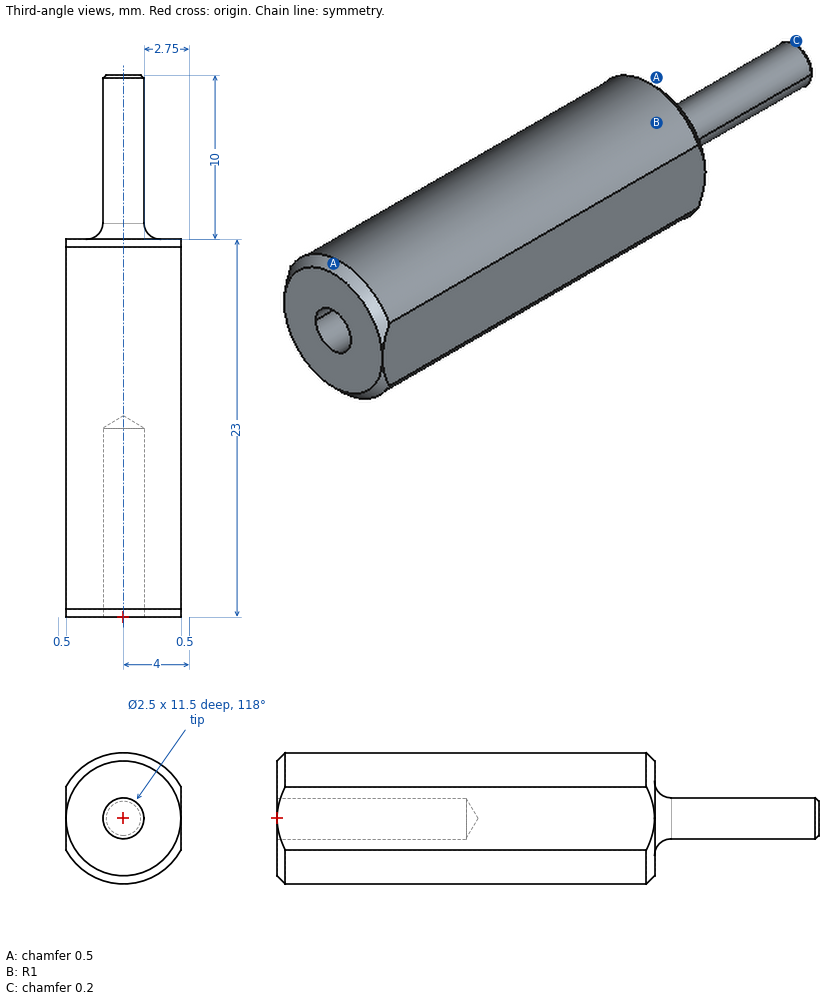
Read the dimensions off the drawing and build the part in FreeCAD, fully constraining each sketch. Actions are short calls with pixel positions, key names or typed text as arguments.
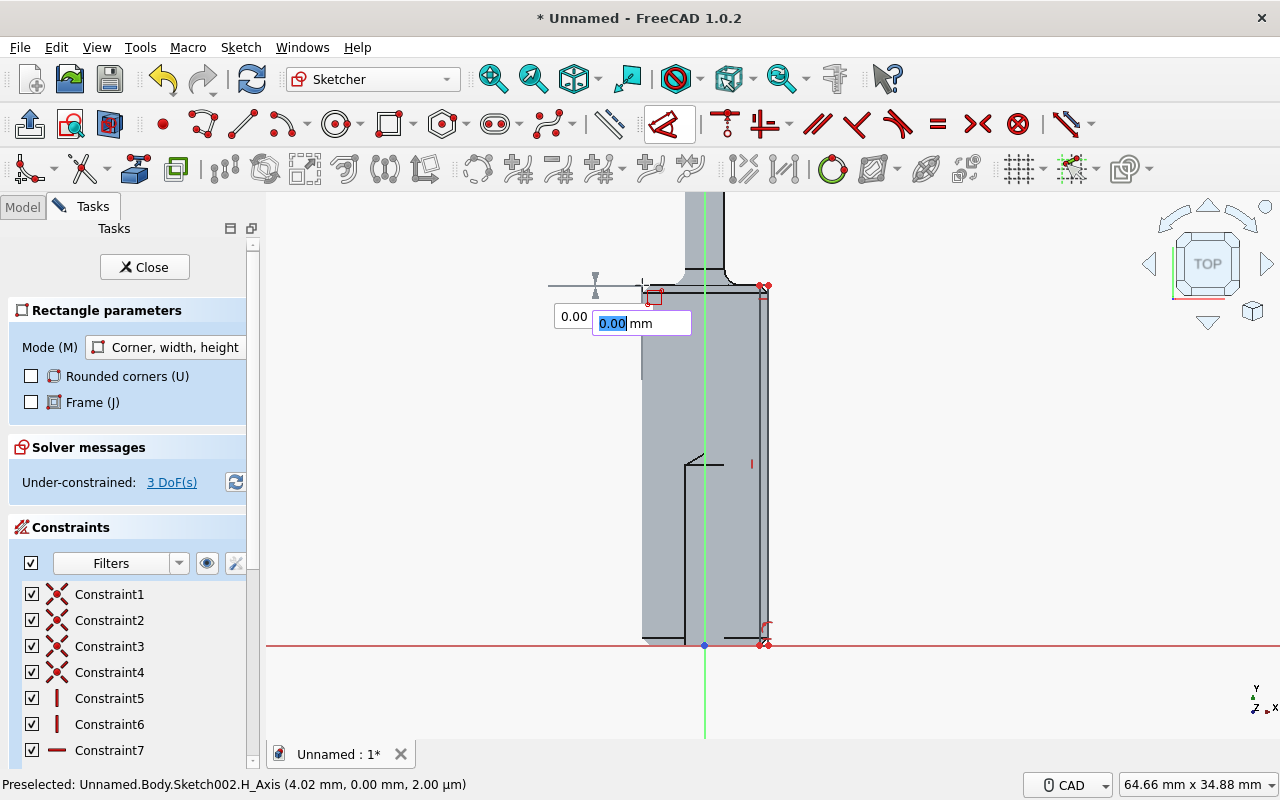
click(650, 646)
key(Escape)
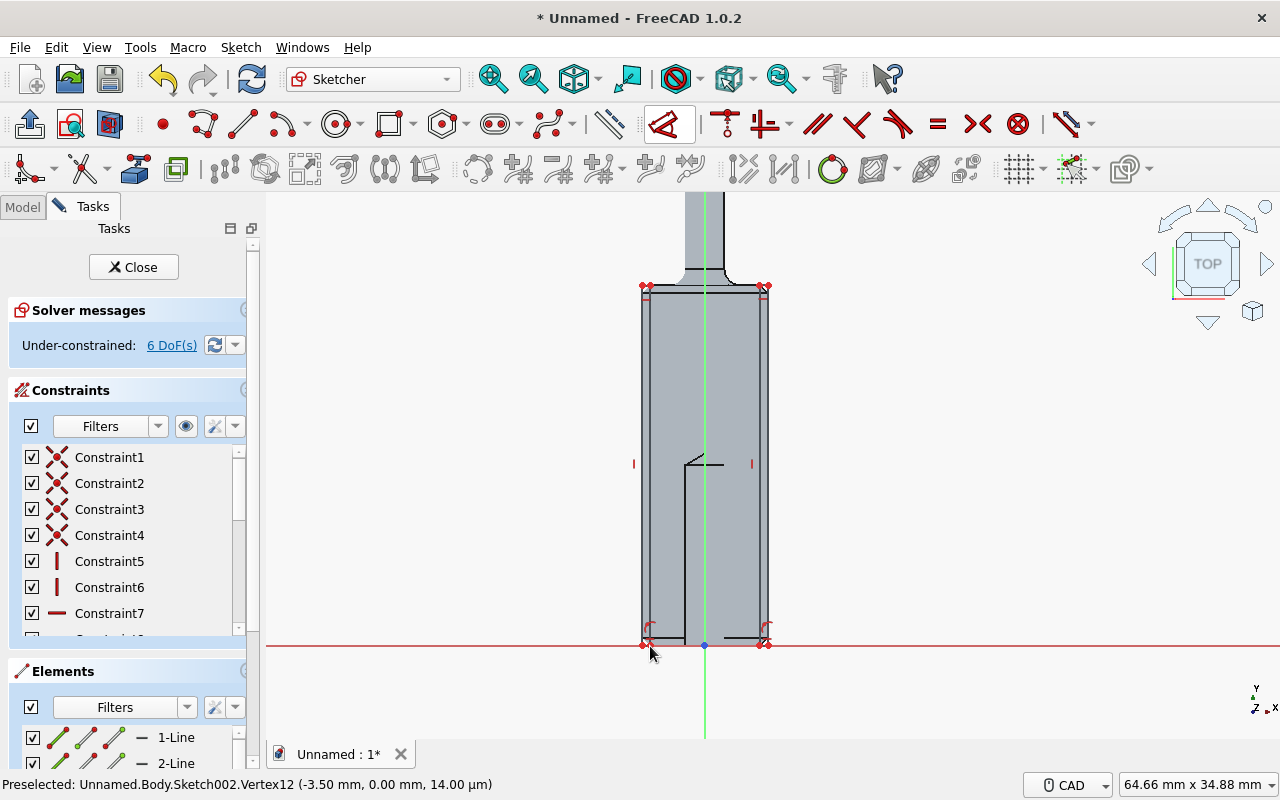
scroll(768, 285, up, 3)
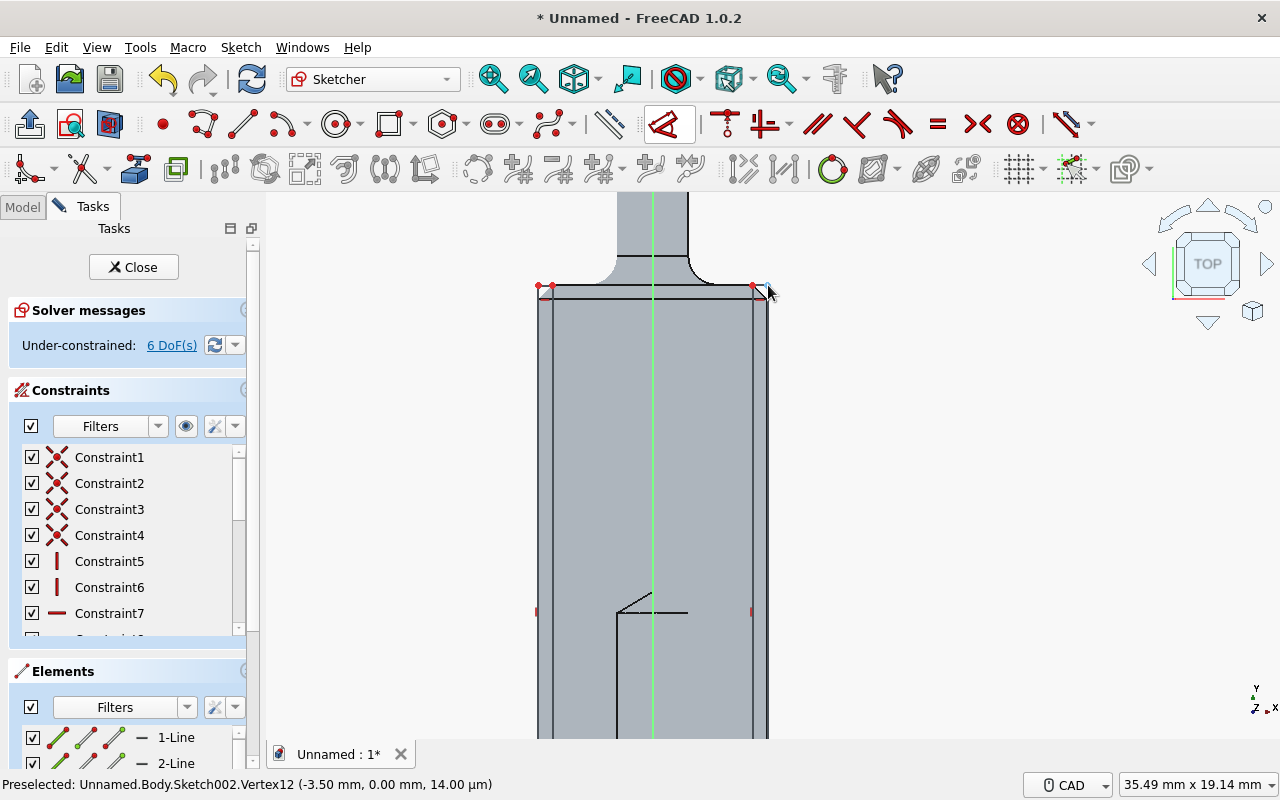
click(768, 285)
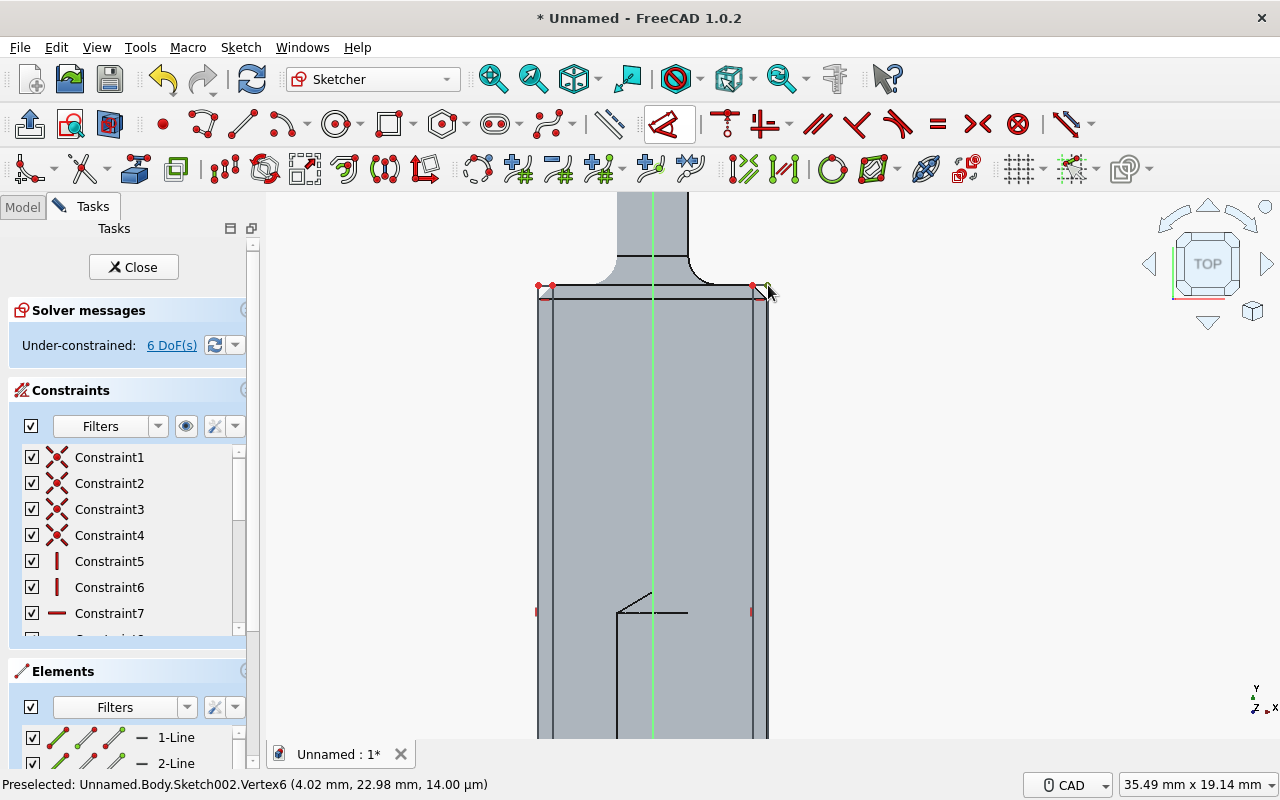
click(538, 286)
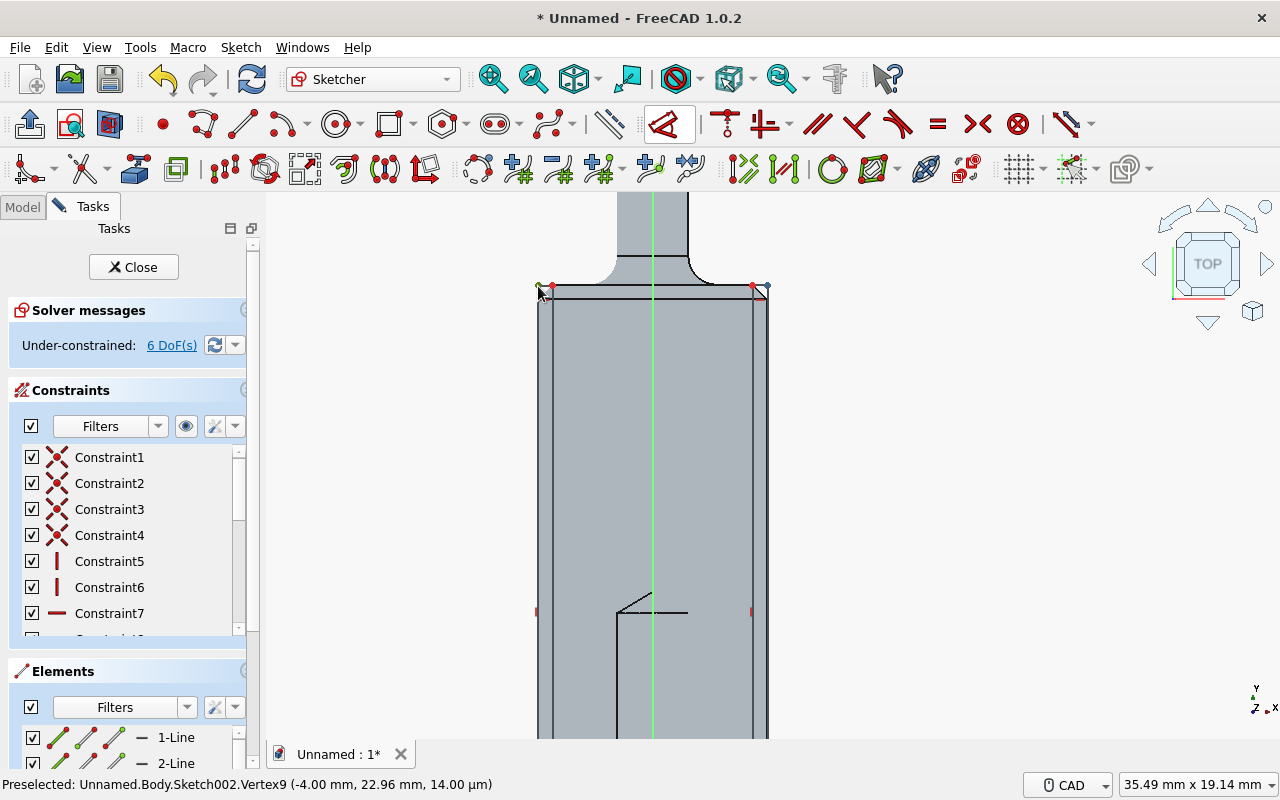
click(653, 676)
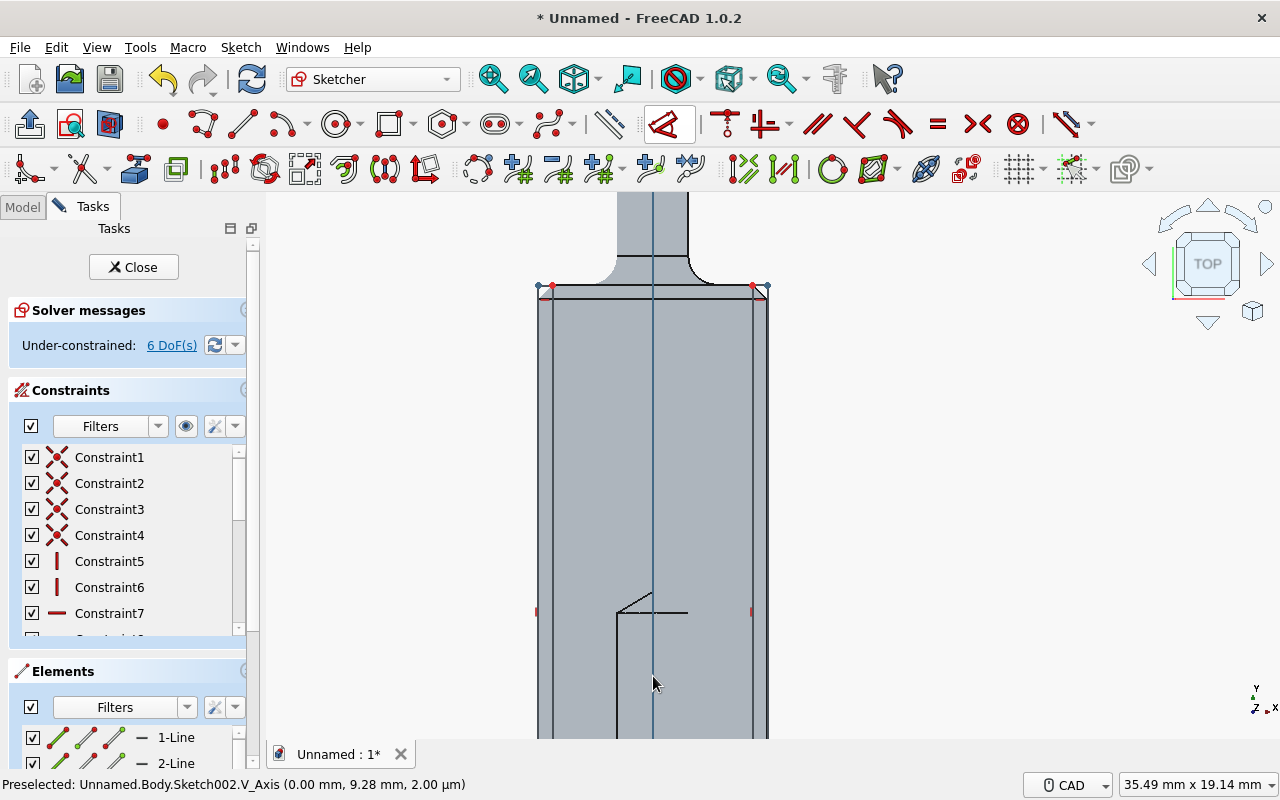
key(s)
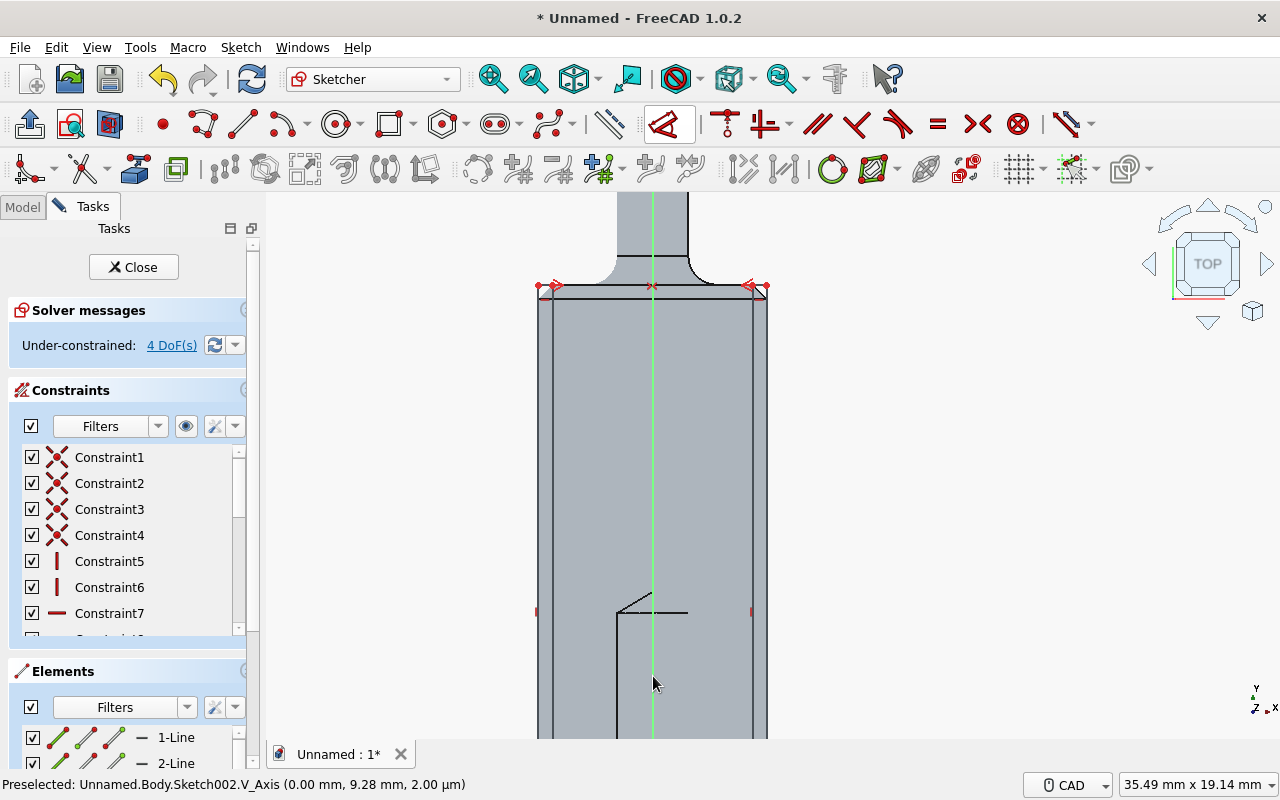
click(753, 482)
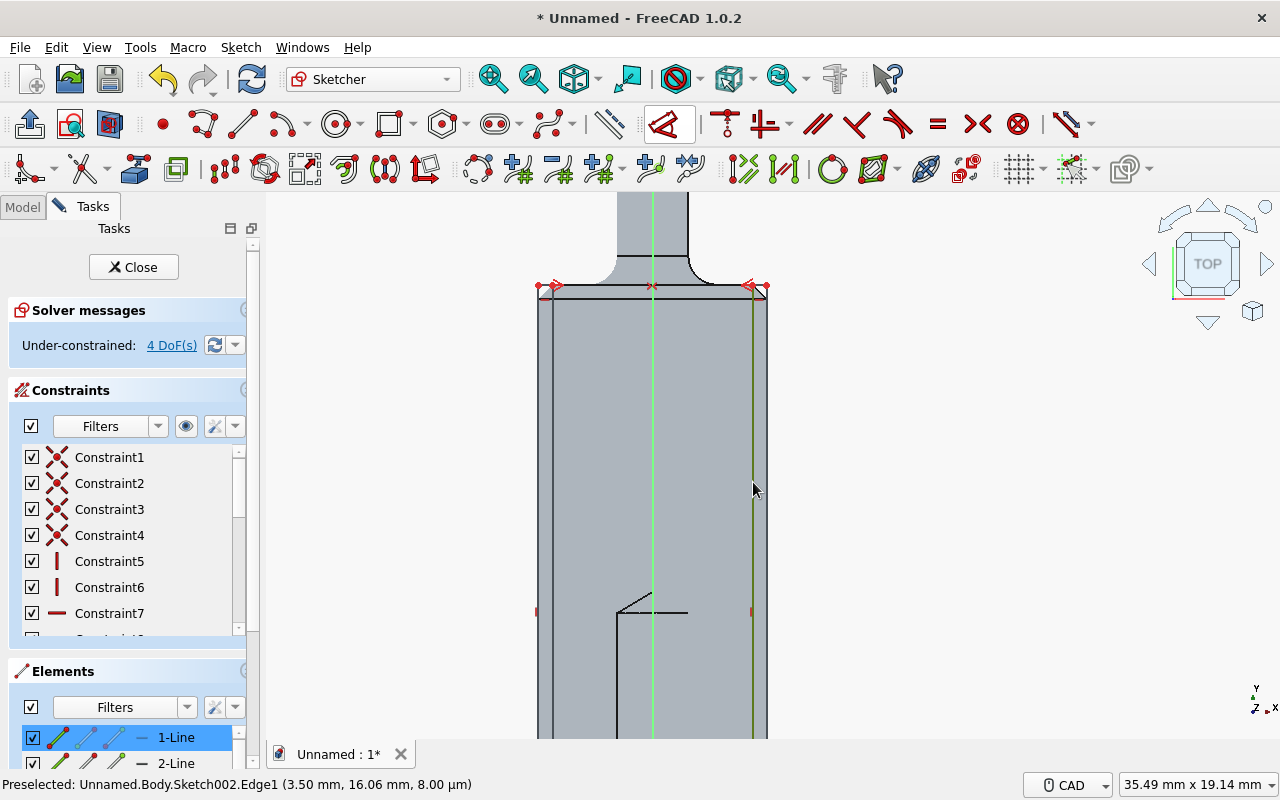
key(i)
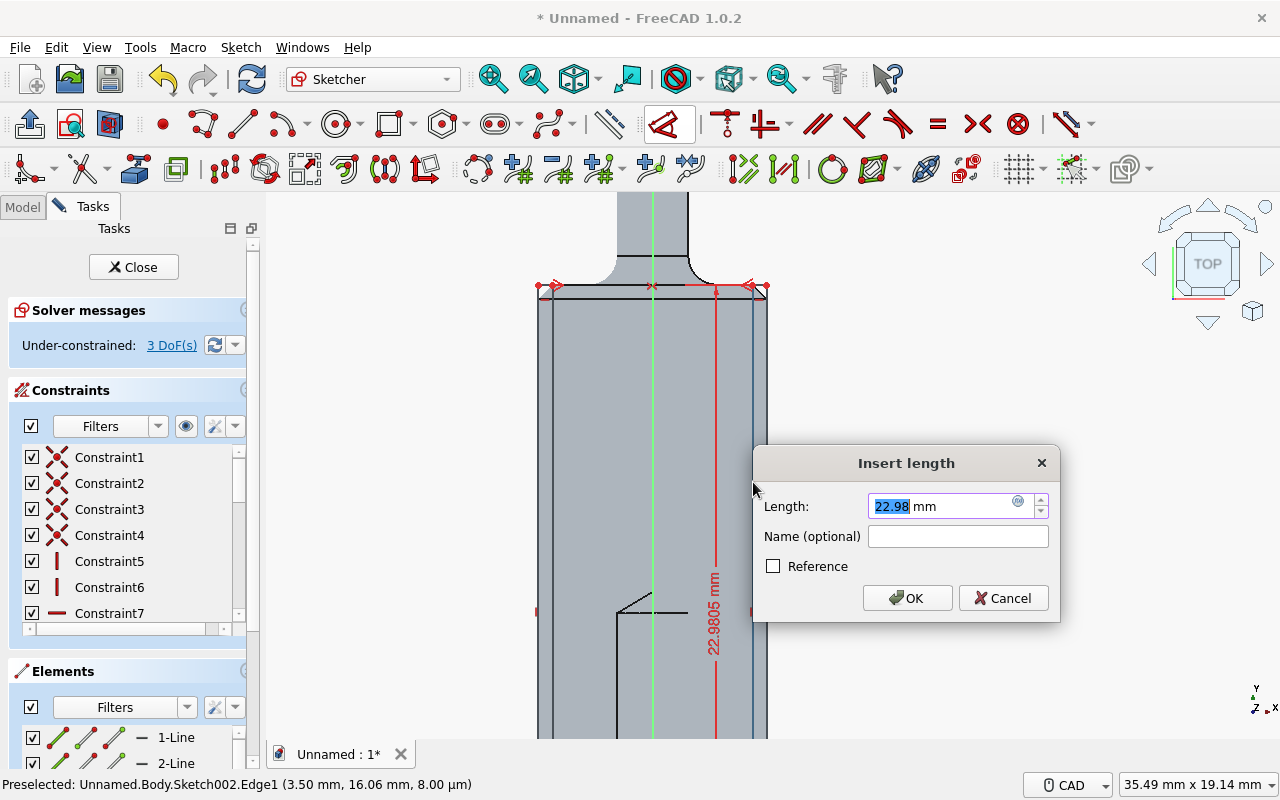
text(23)
key(Return)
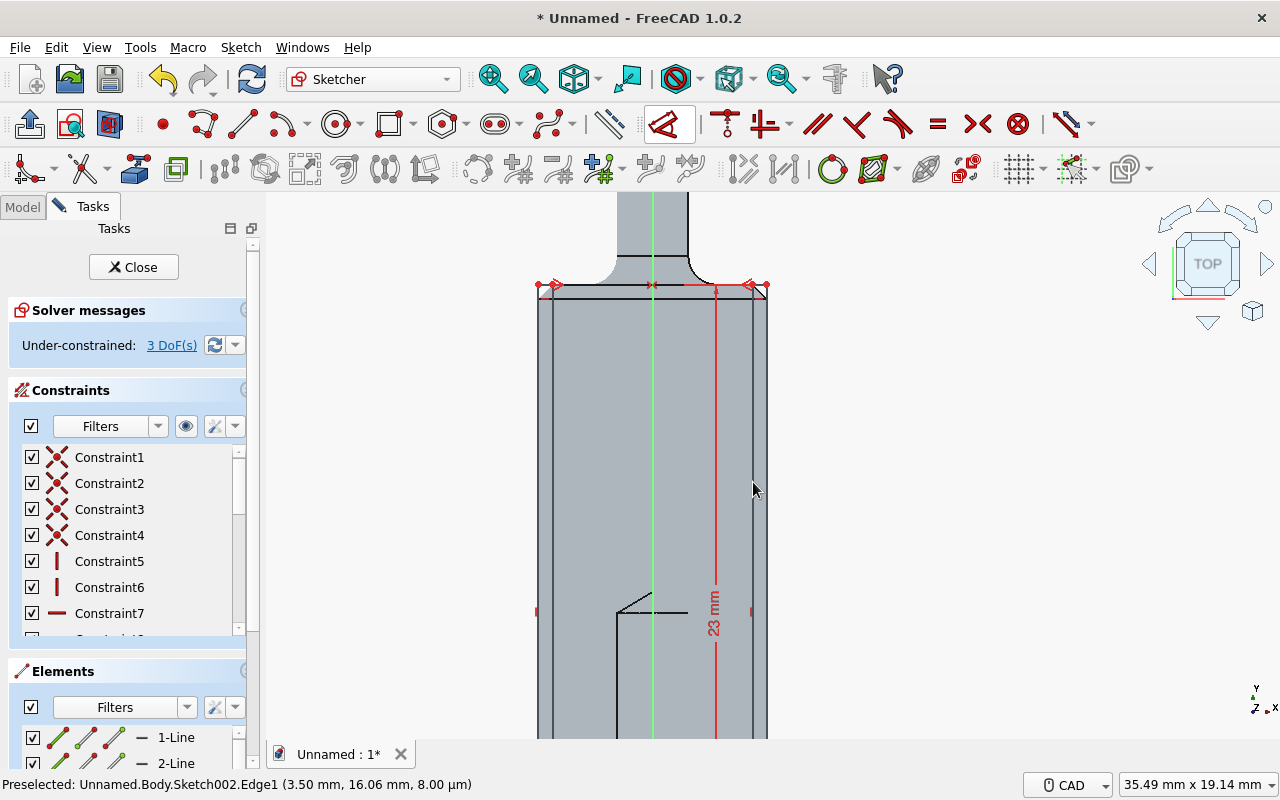
scroll(768, 286, down, 3)